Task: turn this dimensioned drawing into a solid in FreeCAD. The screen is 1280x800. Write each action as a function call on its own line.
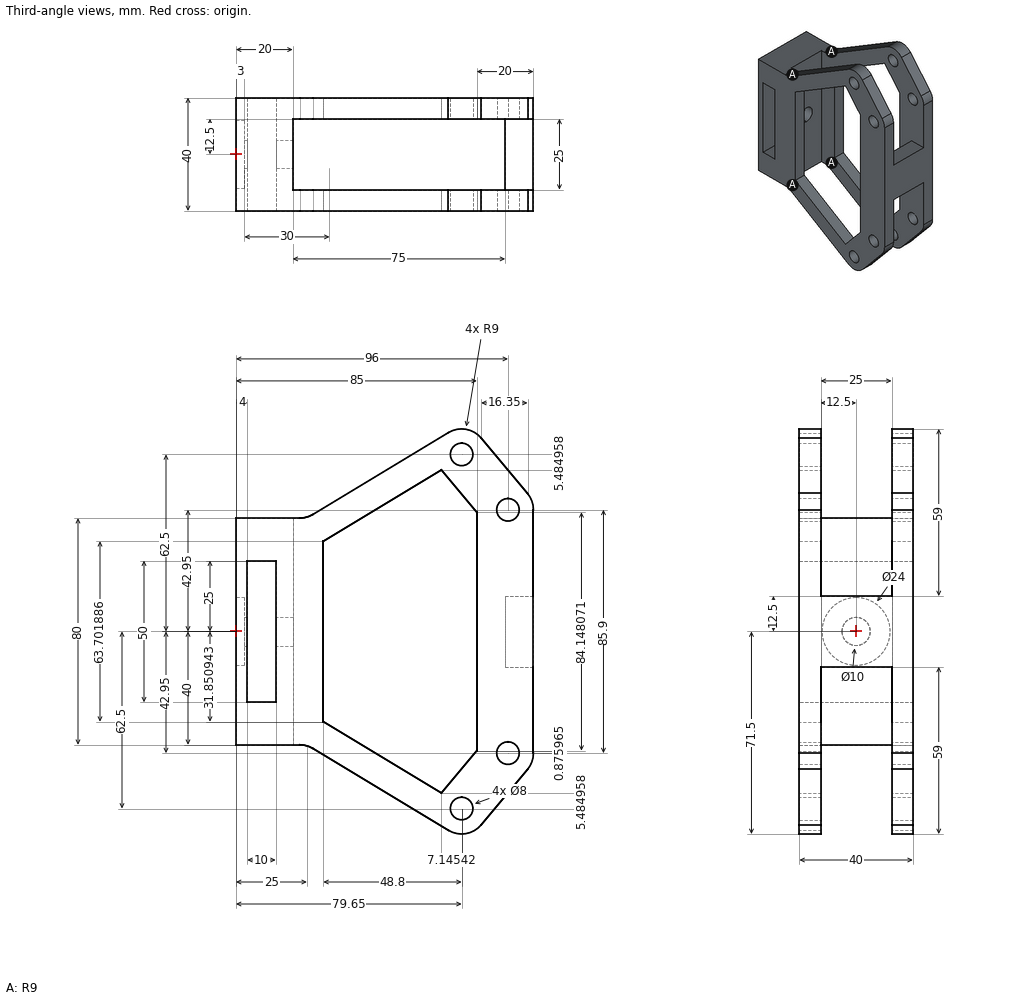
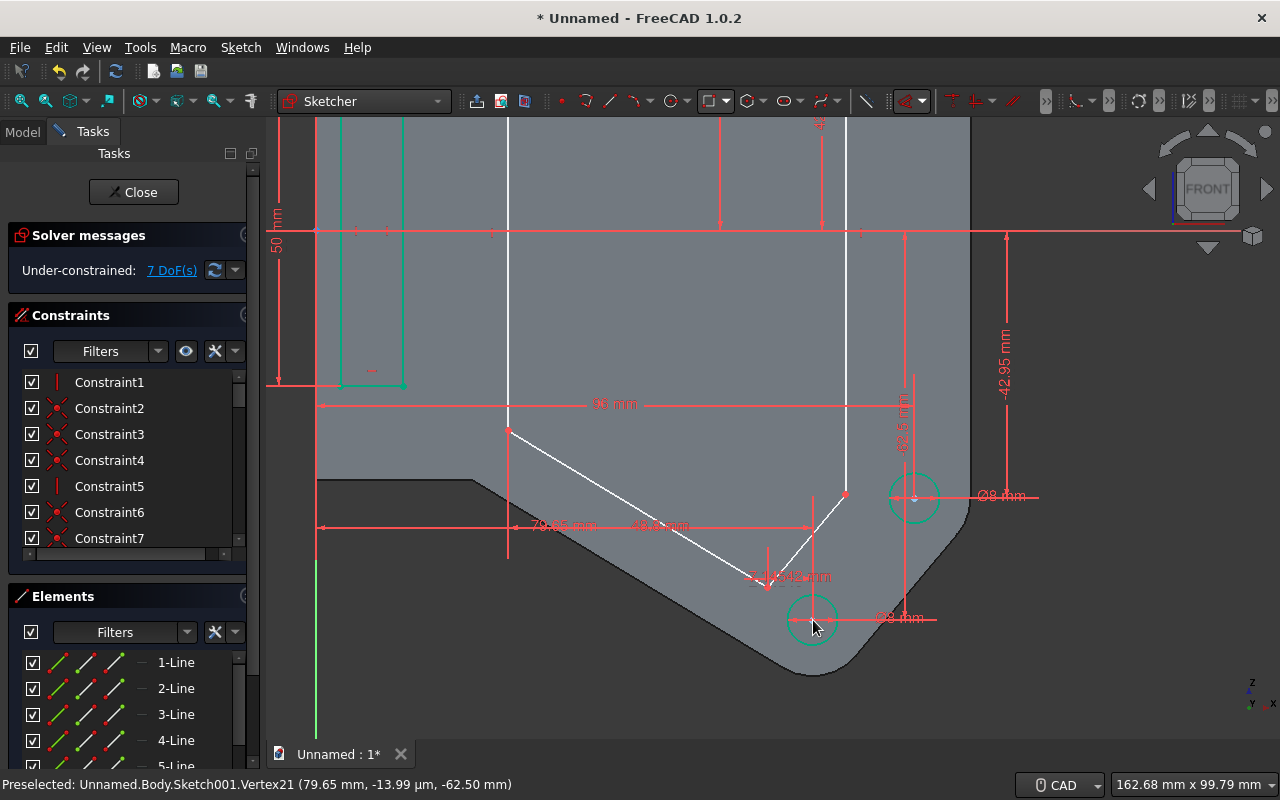
scroll(767, 589, down, 4)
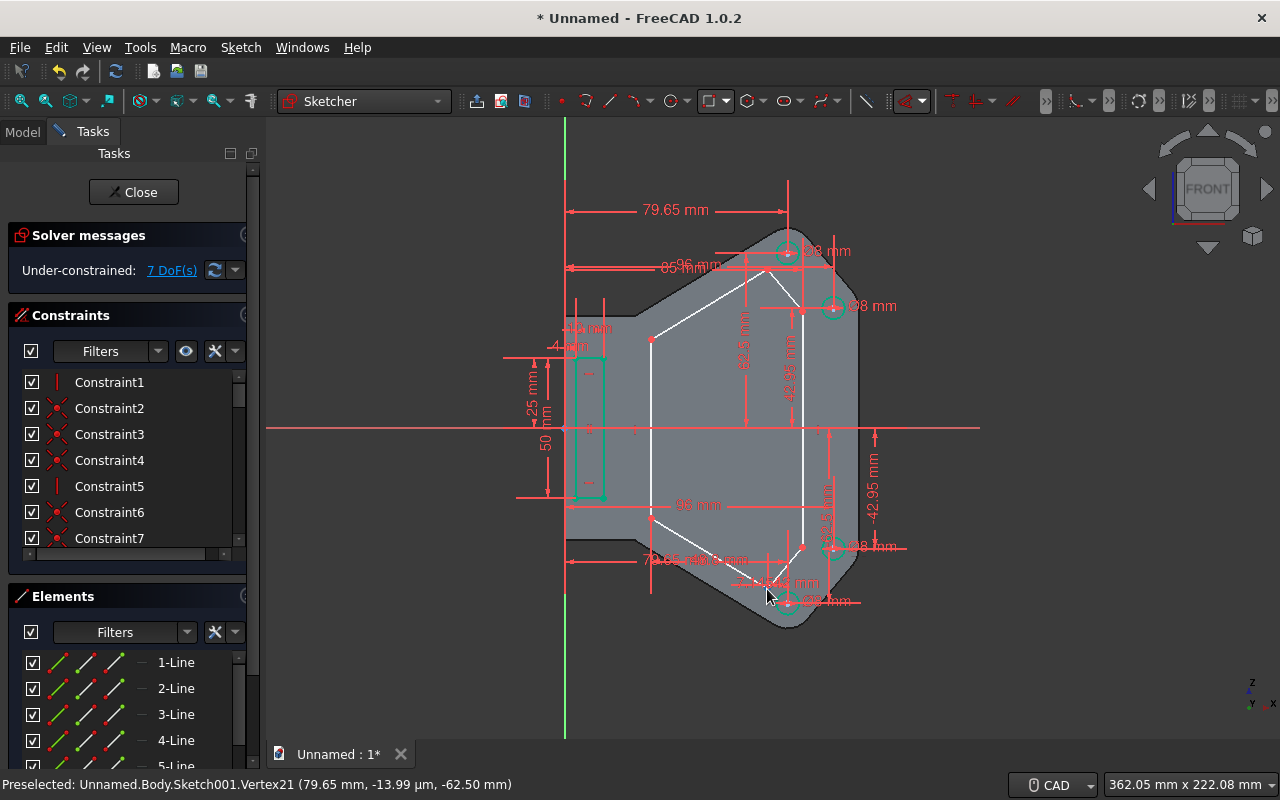
scroll(767, 270, up, 4)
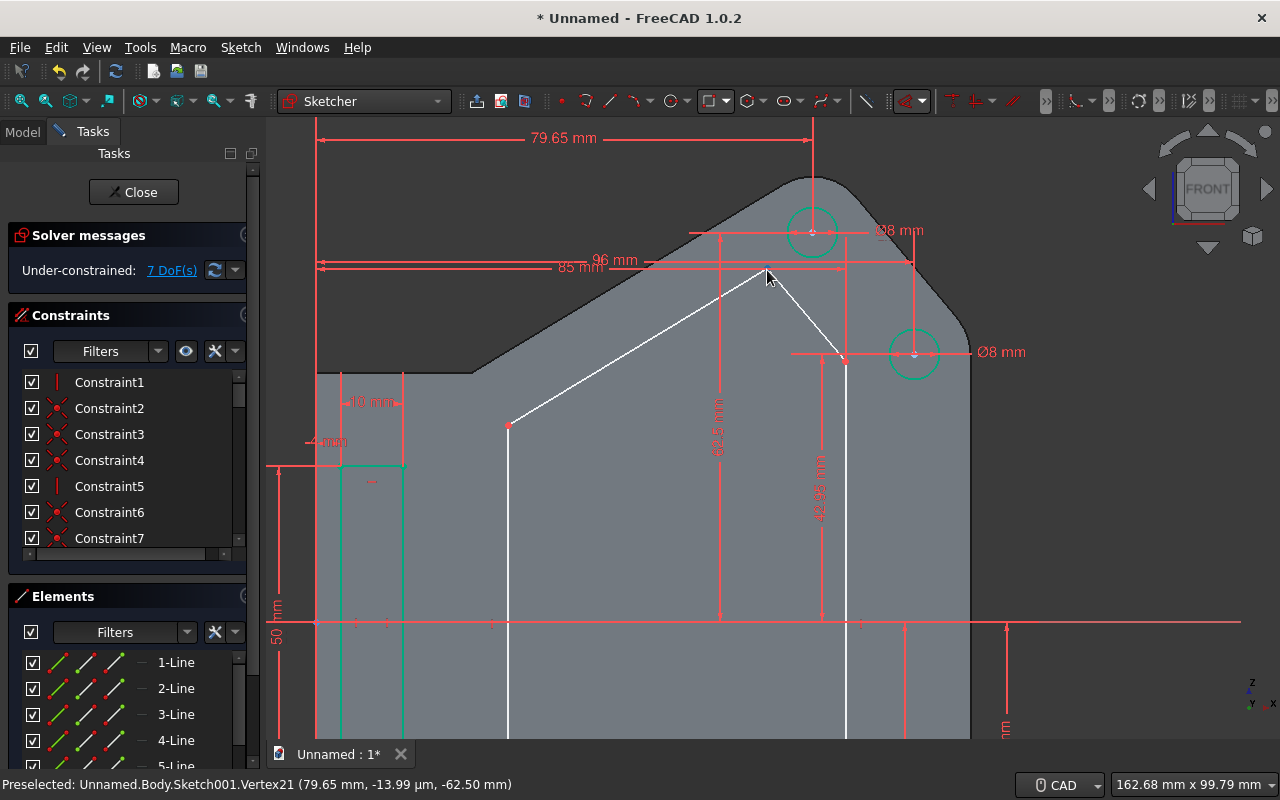
click(767, 269)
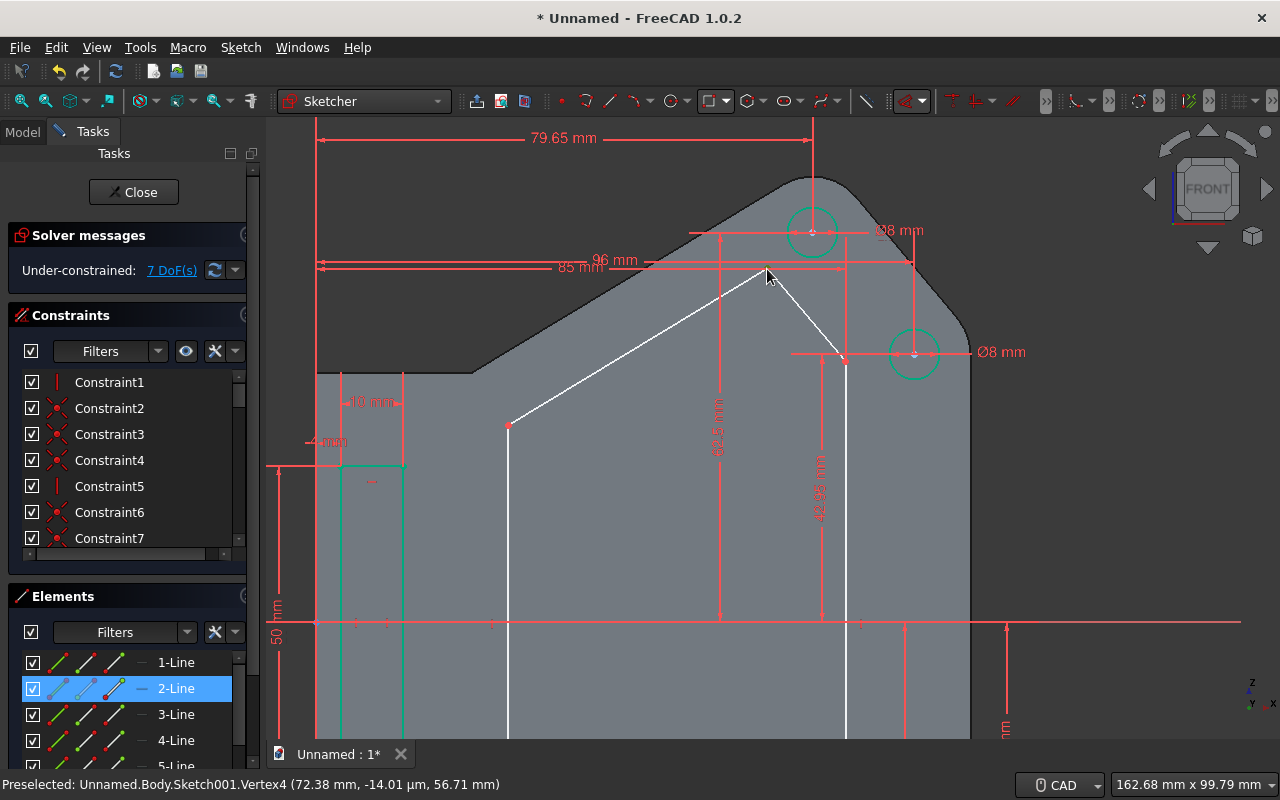
click(813, 233)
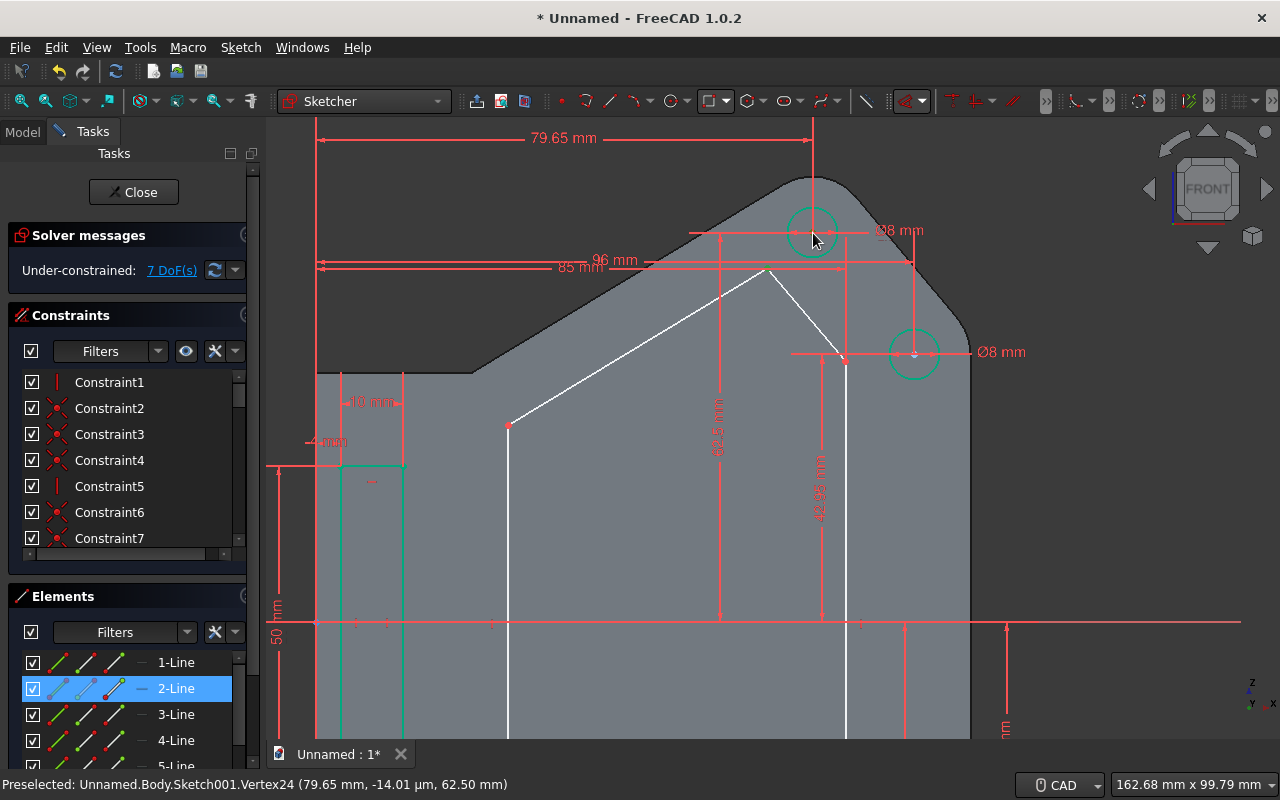
key(l)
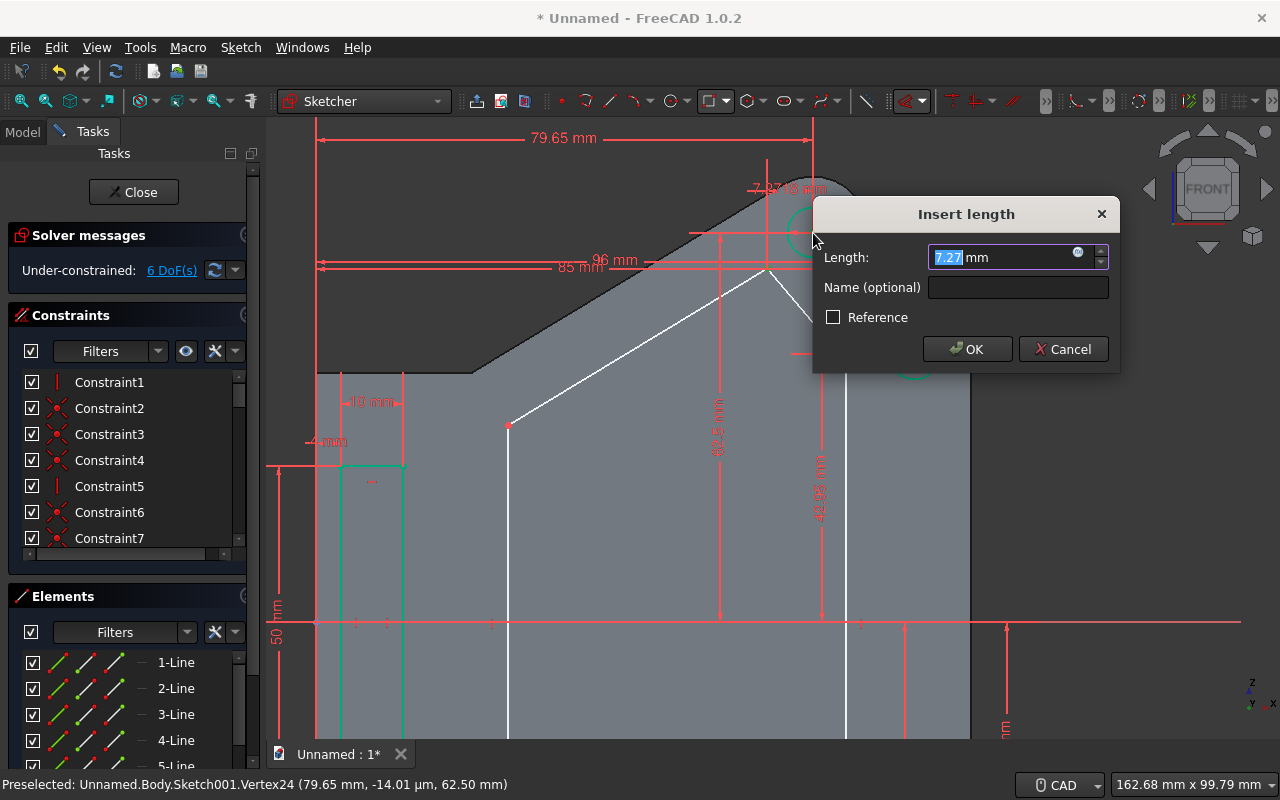
text(7.14542)
key(Return)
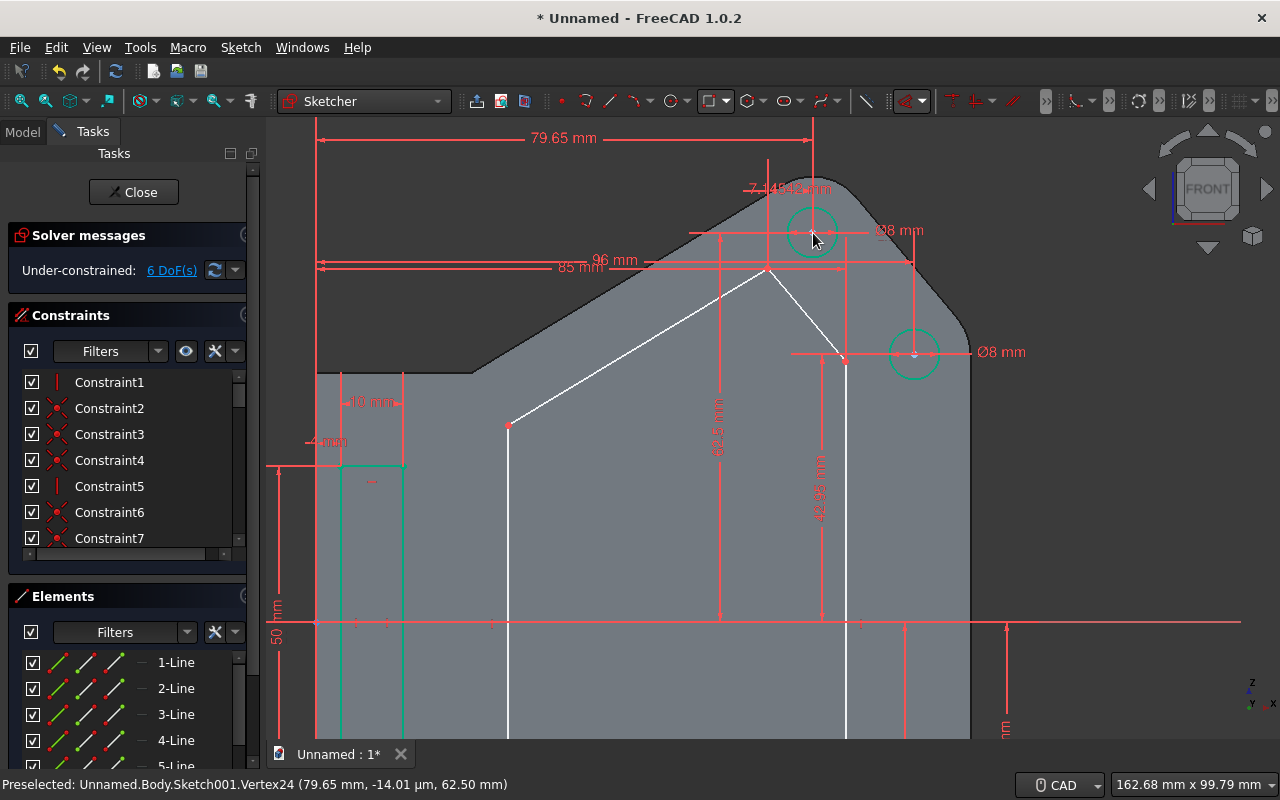
click(508, 703)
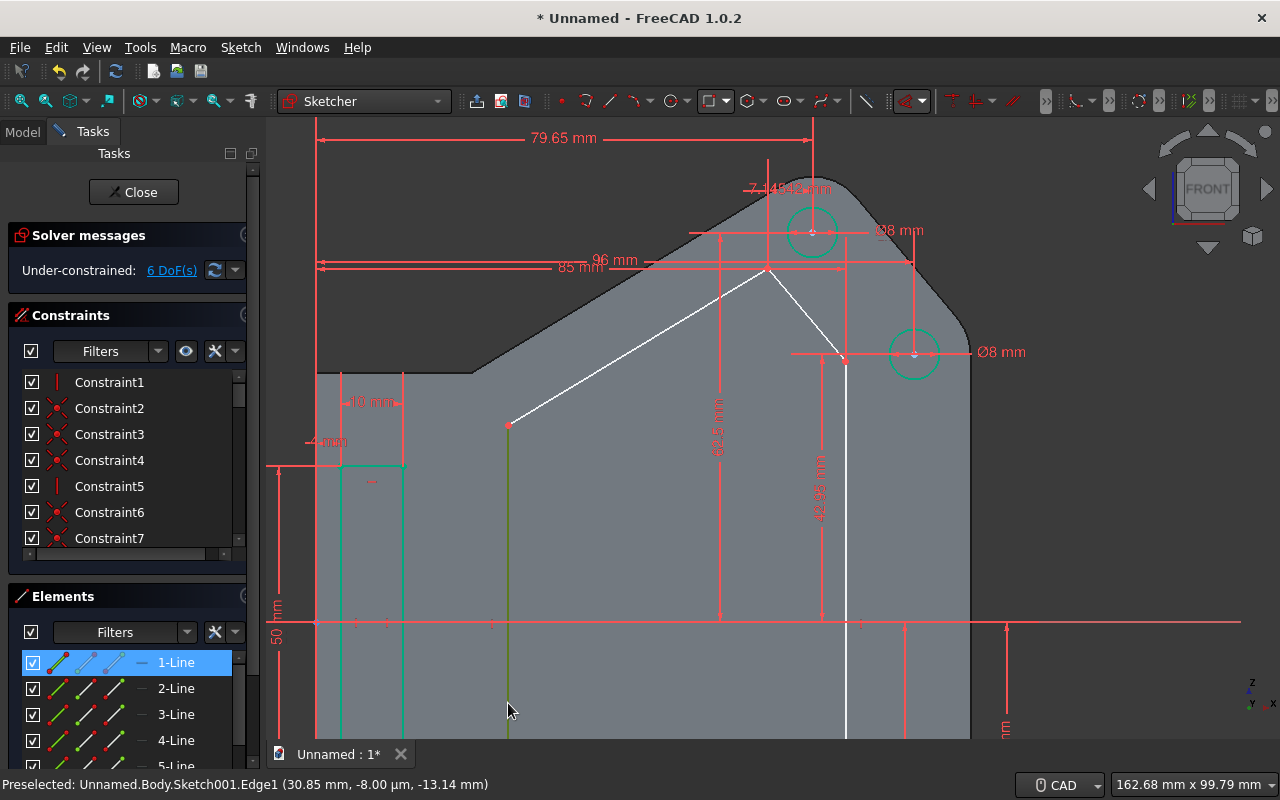
key(i)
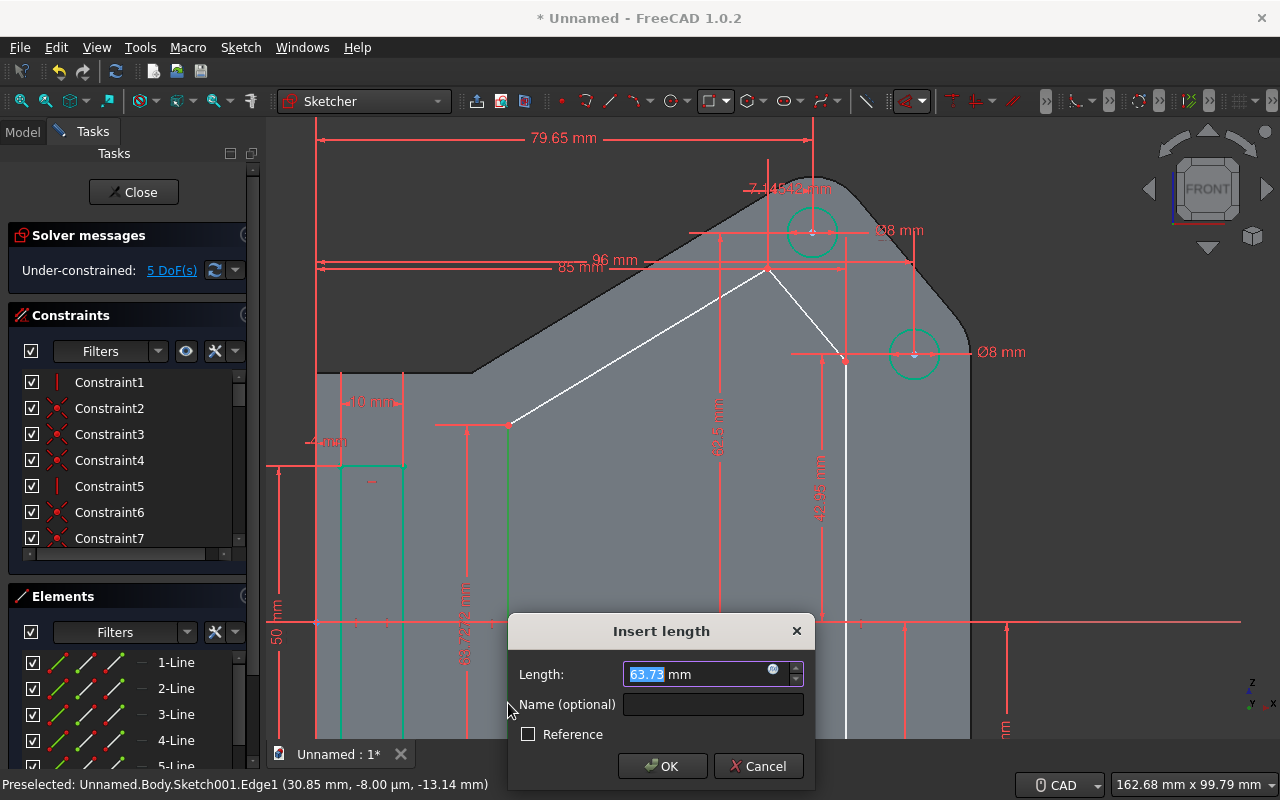
text(63.701886)
key(Return)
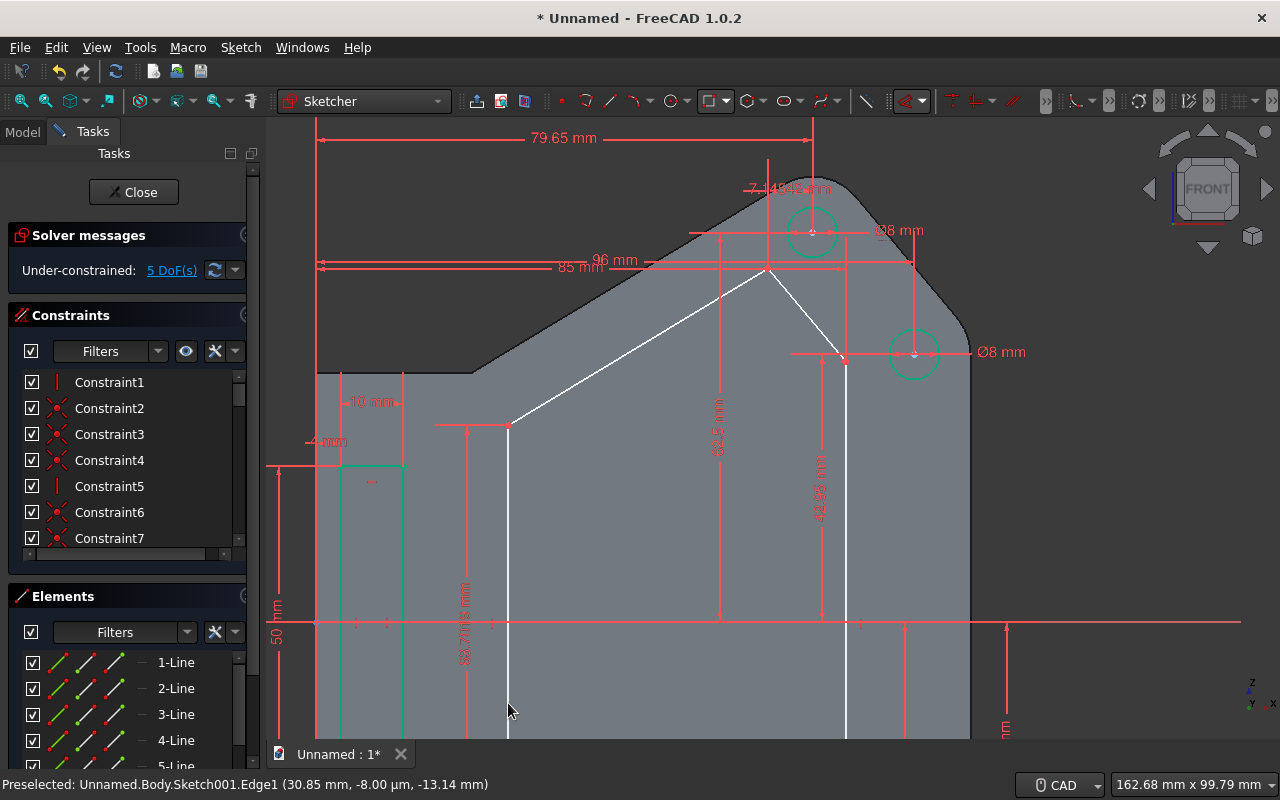
click(846, 519)